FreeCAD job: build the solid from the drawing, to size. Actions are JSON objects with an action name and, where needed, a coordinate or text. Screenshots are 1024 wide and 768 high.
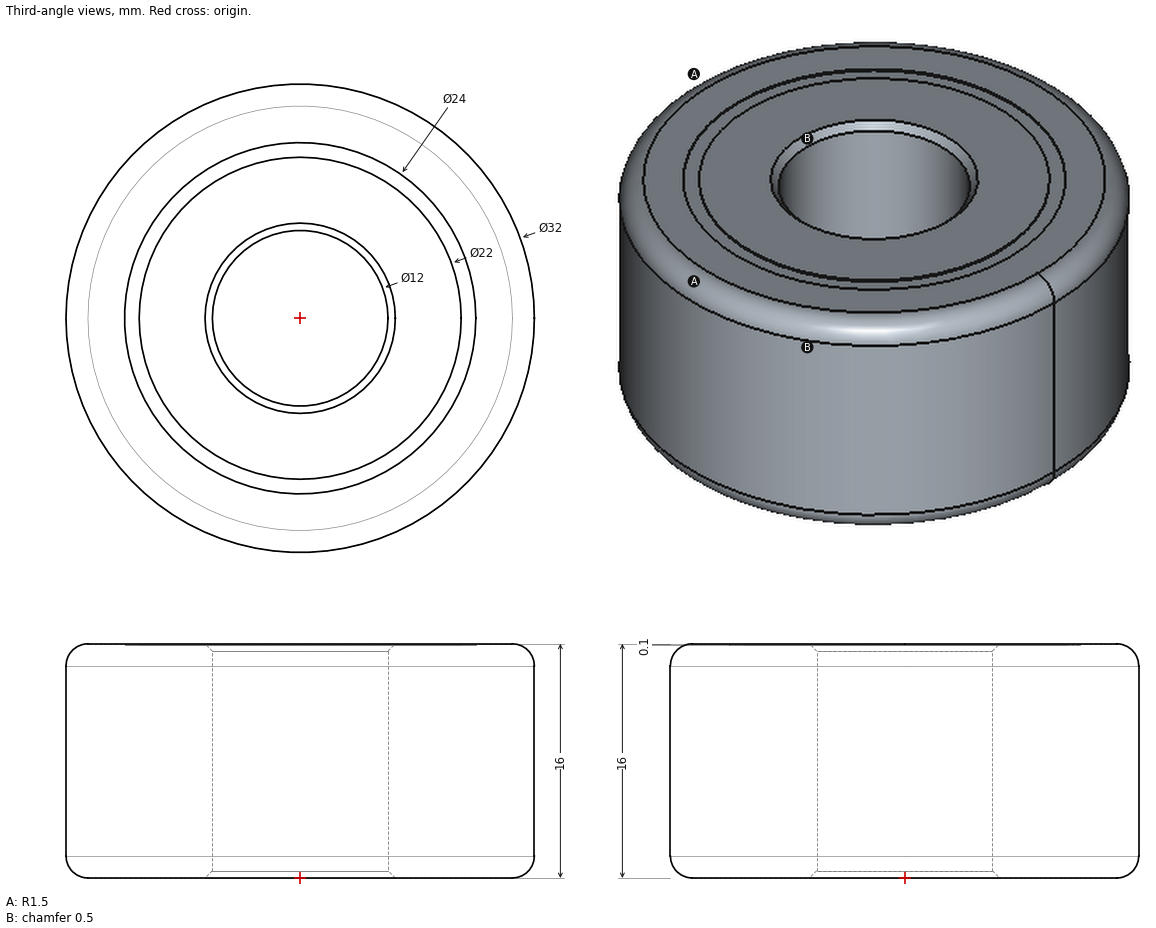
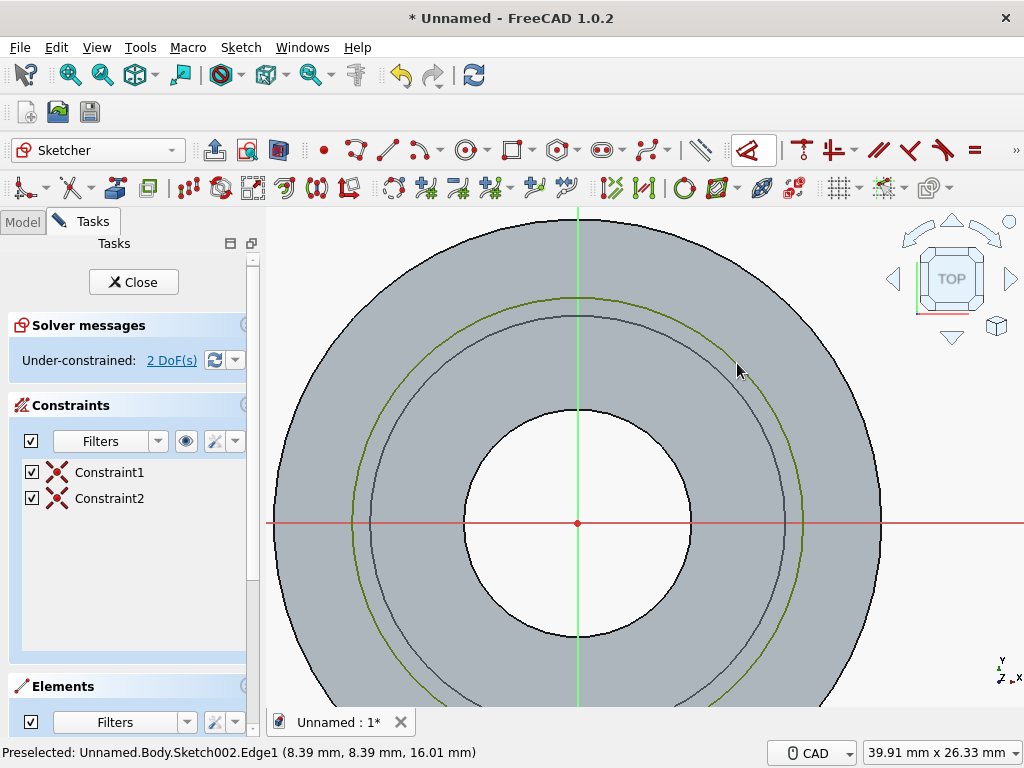
{"action": "key", "text": "k o"}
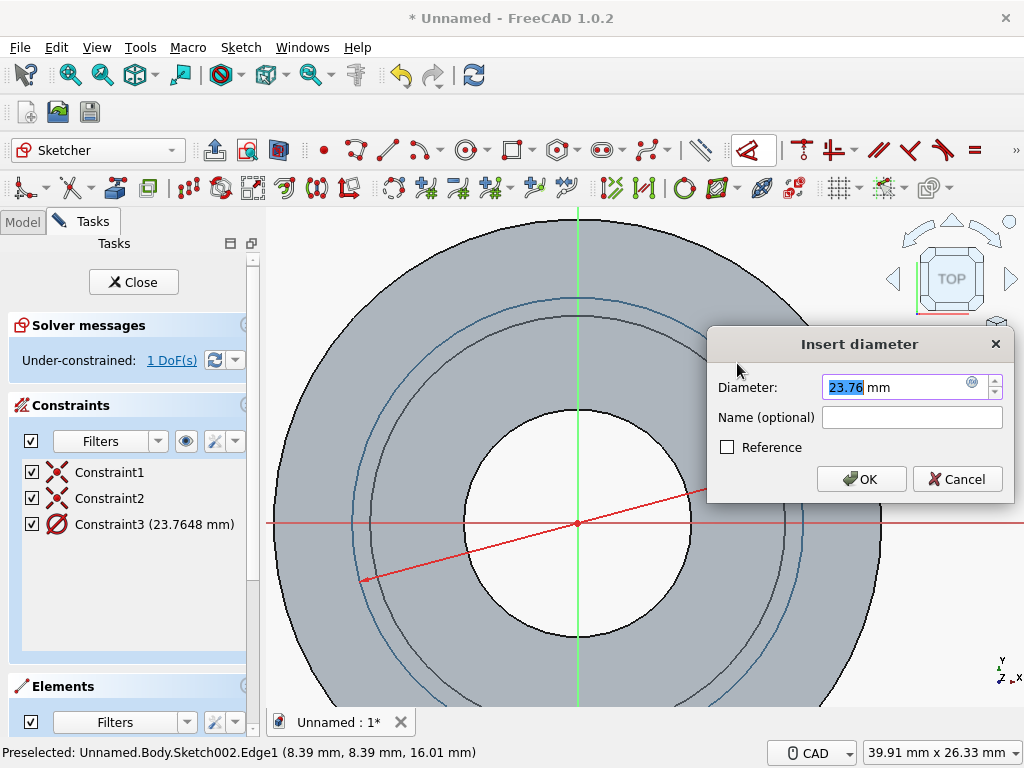
{"action": "type", "text": "24"}
{"action": "key", "text": "Return"}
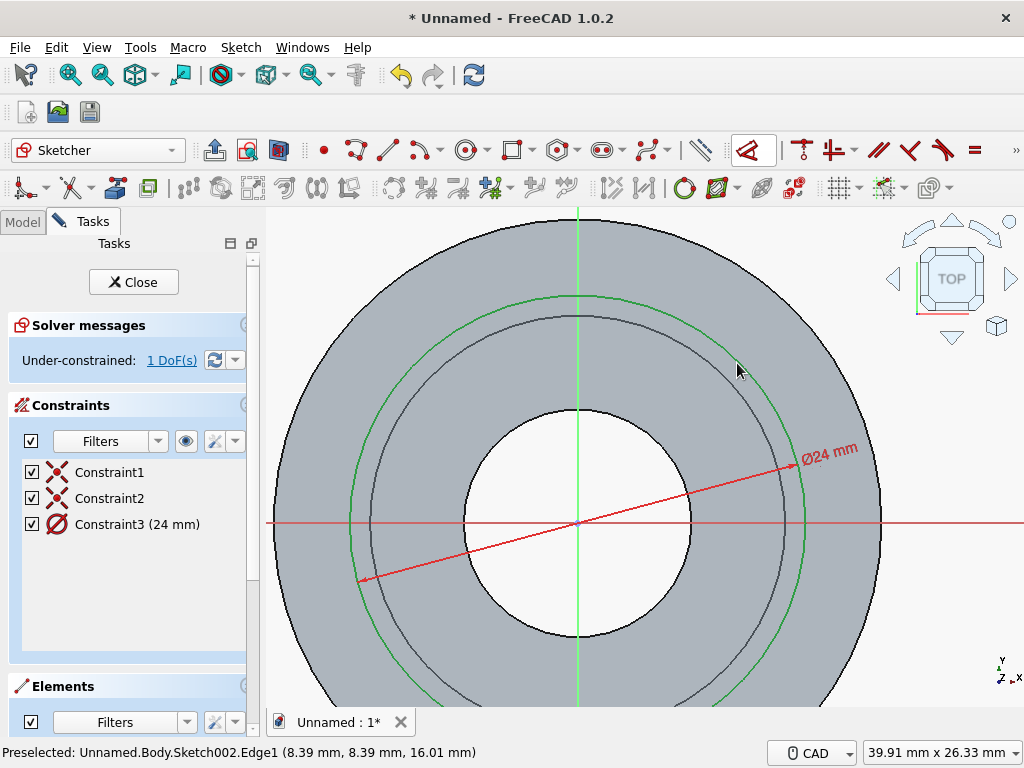
{"action": "left_click", "coordinate": [724, 376]}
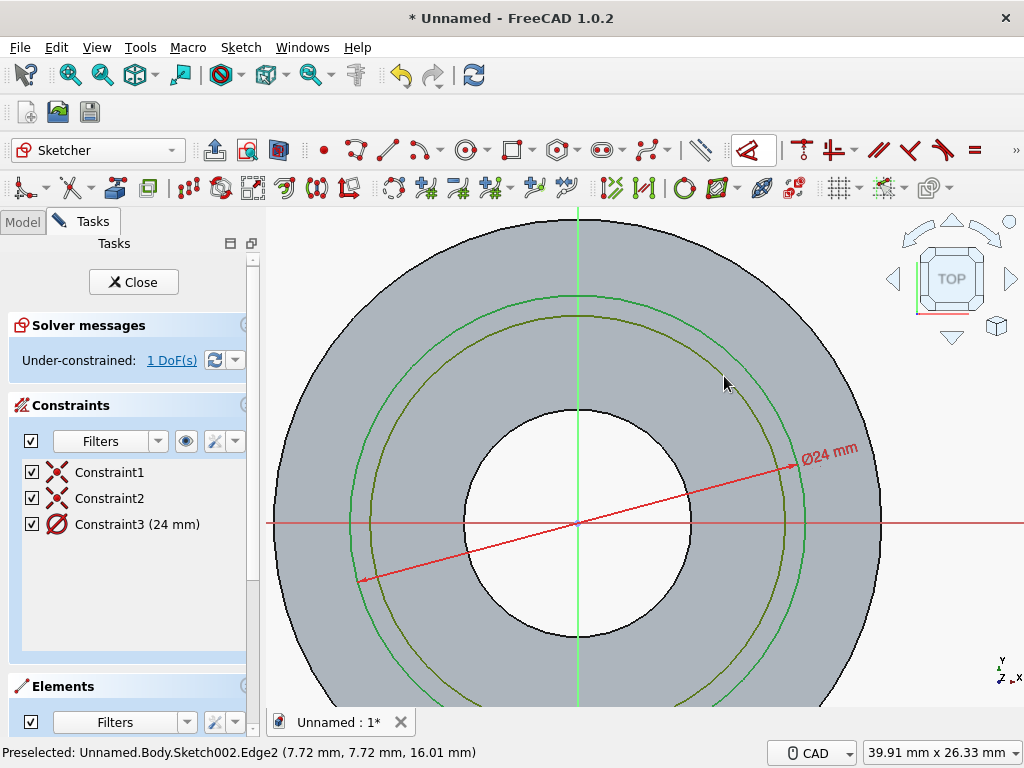
{"action": "left_click", "coordinate": [770, 150]}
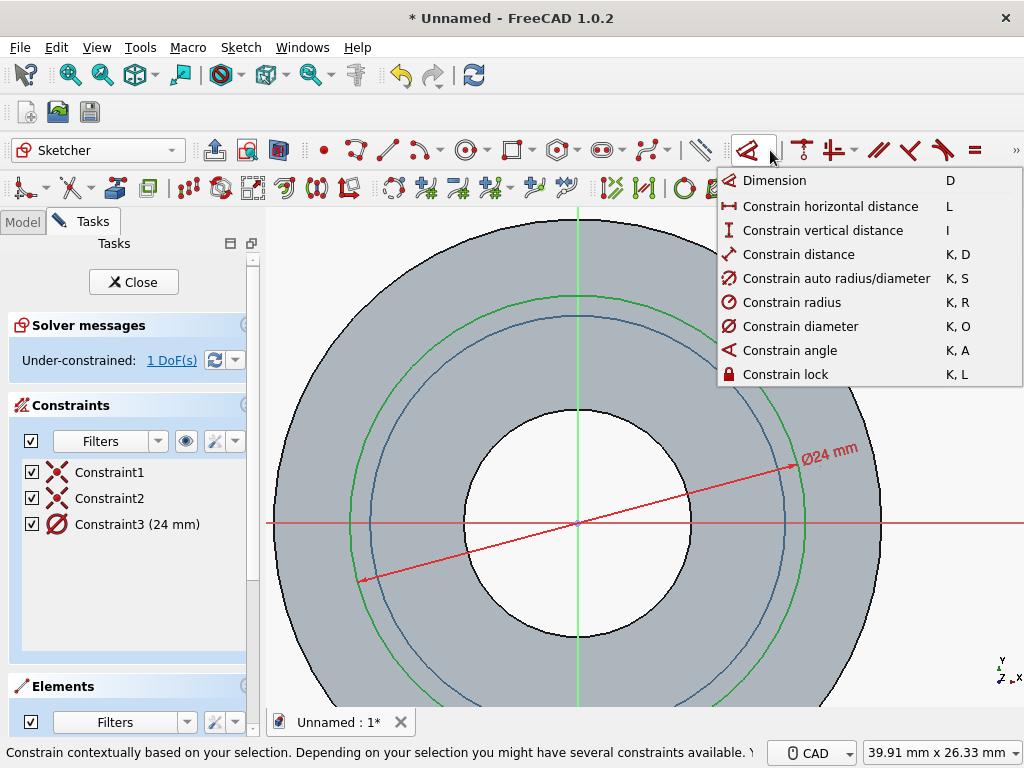
{"action": "left_click", "coordinate": [870, 326]}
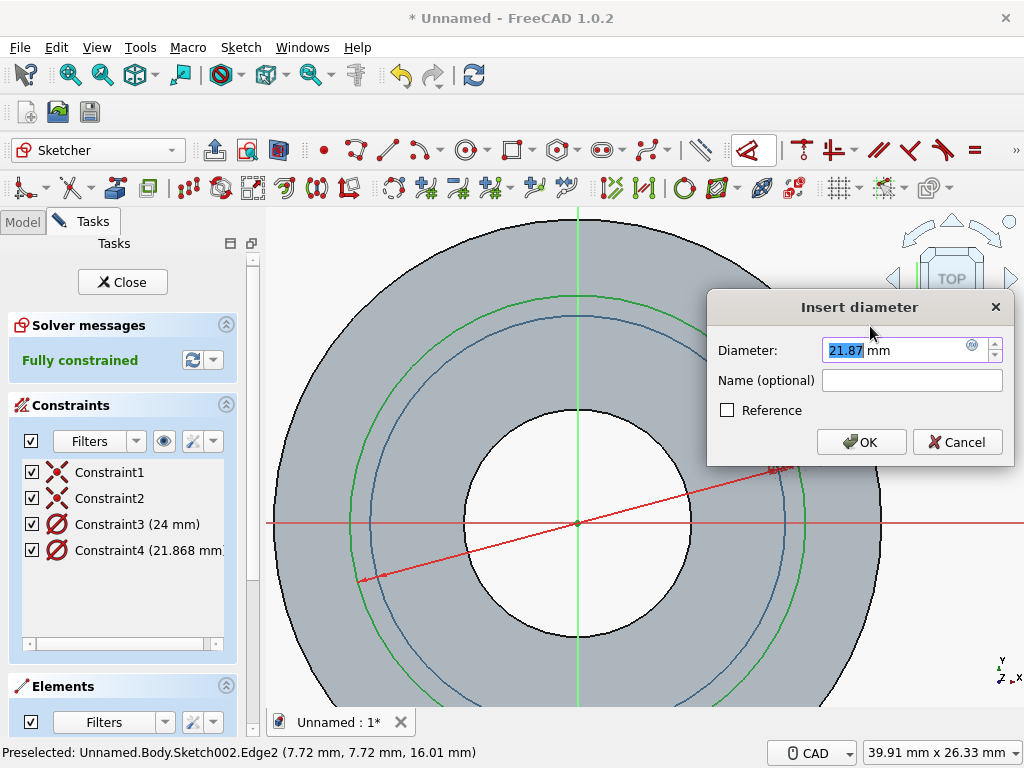
{"action": "type", "text": "22"}
{"action": "key", "text": "Return"}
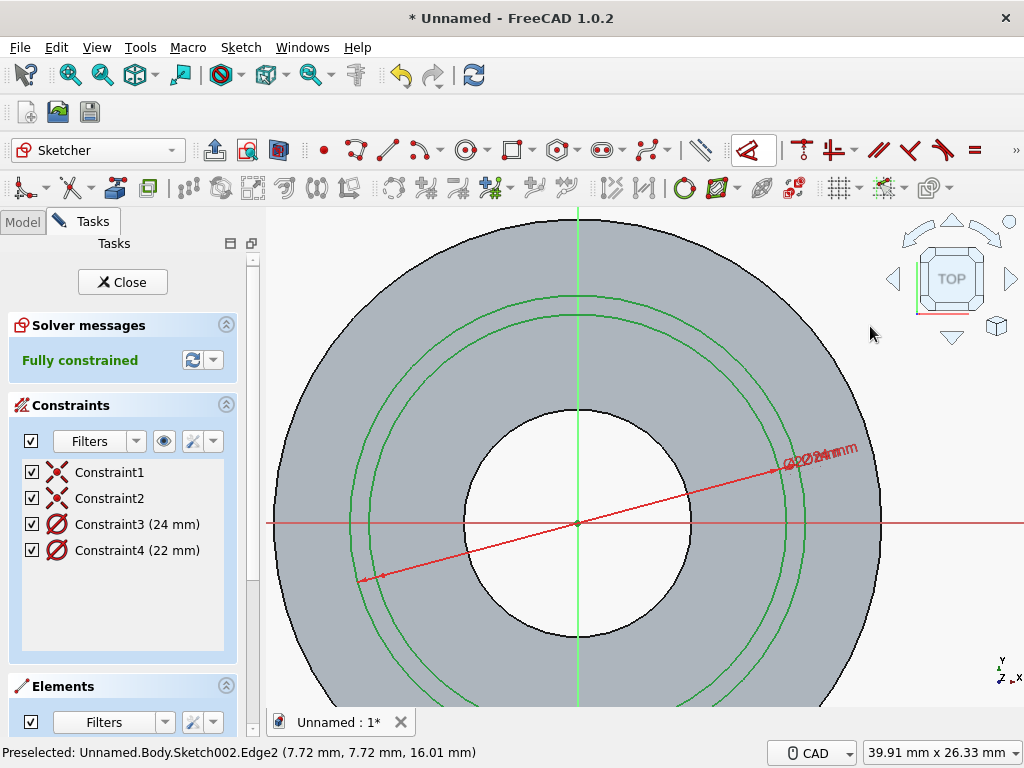
{"action": "left_click", "coordinate": [123, 282]}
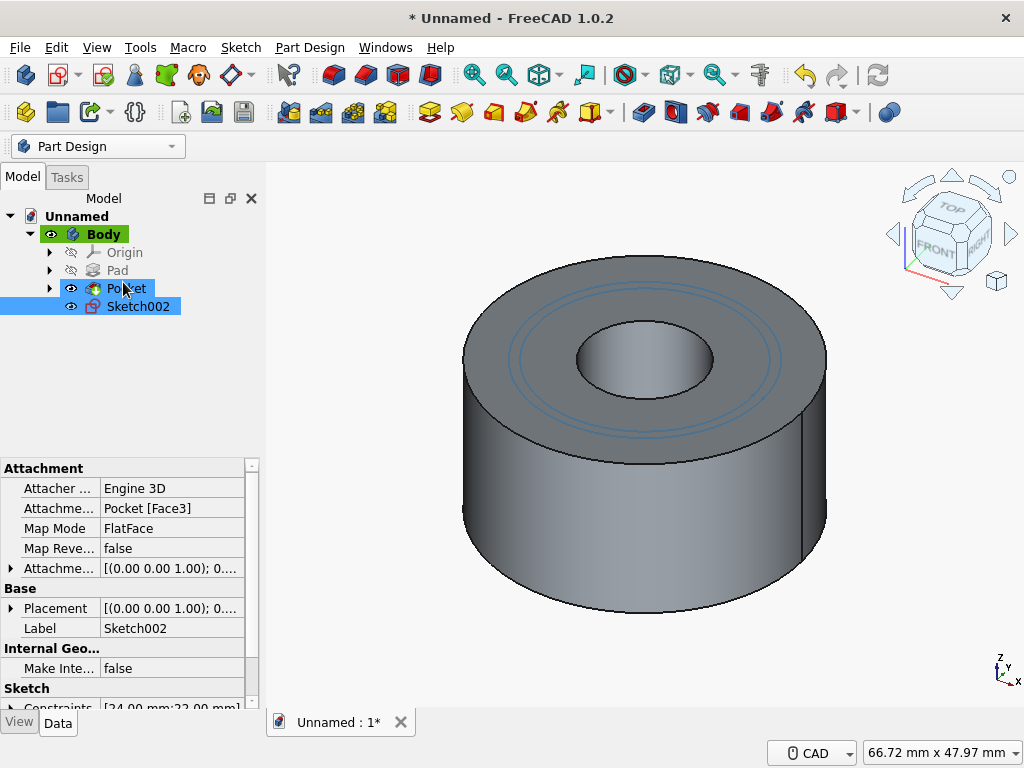
{"action": "left_click", "coordinate": [644, 112]}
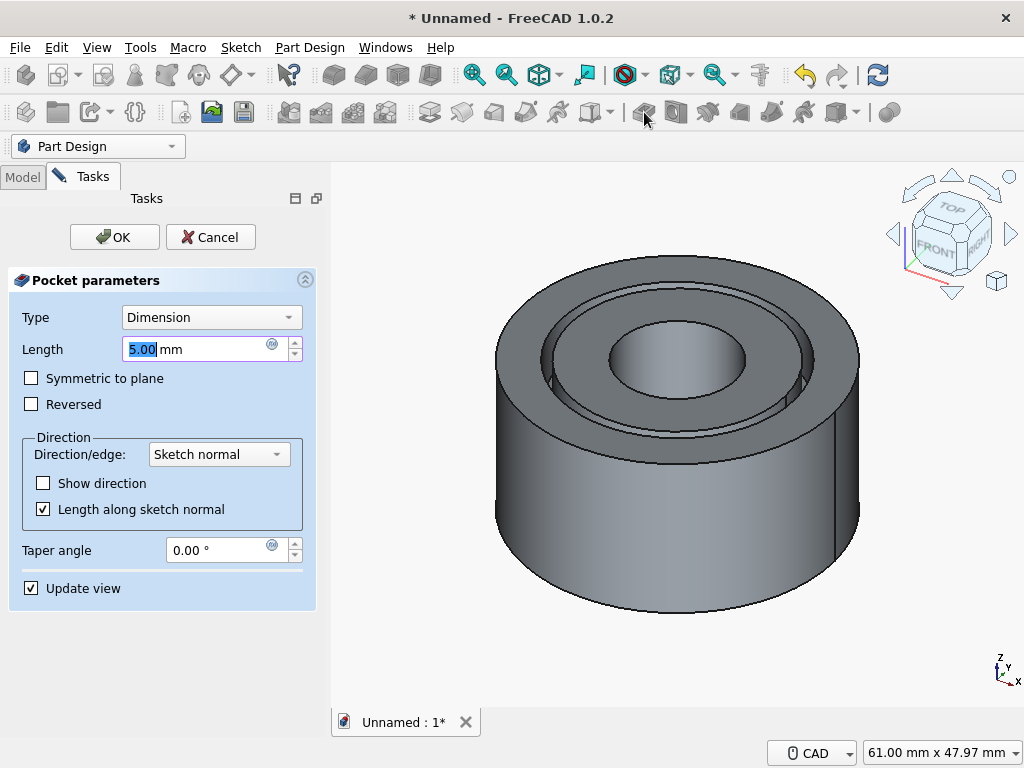
{"action": "type", "text": "0.1"}
{"action": "key", "text": "Tab"}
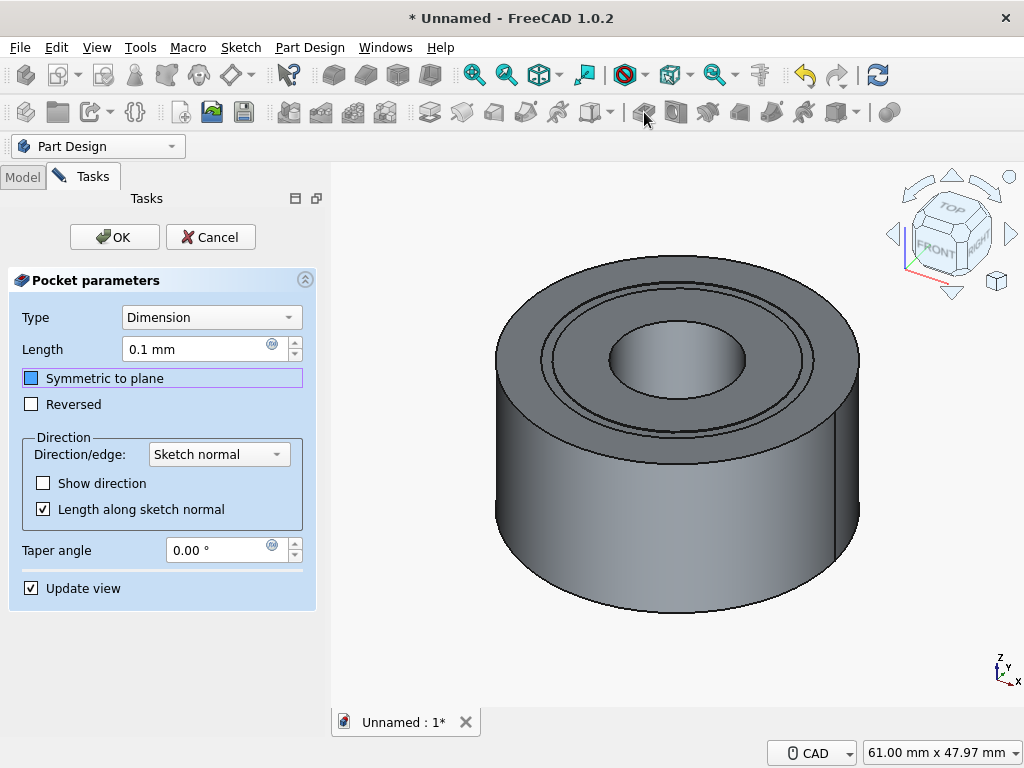
{"action": "left_click", "coordinate": [115, 237]}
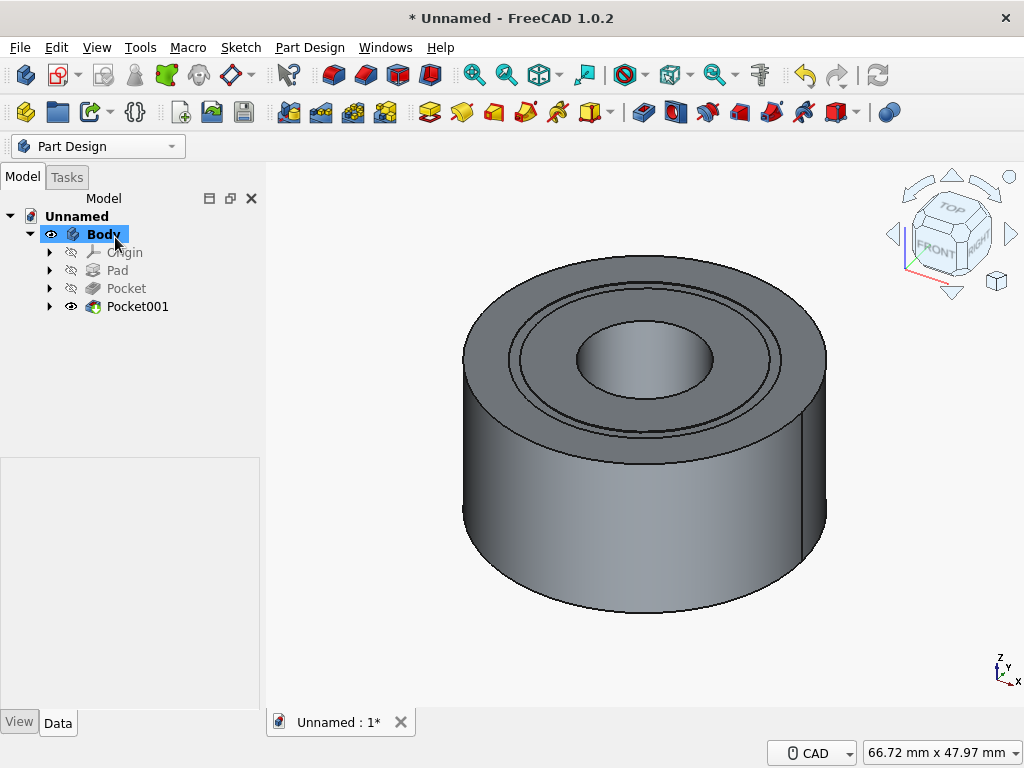
{"action": "left_click", "coordinate": [464, 370]}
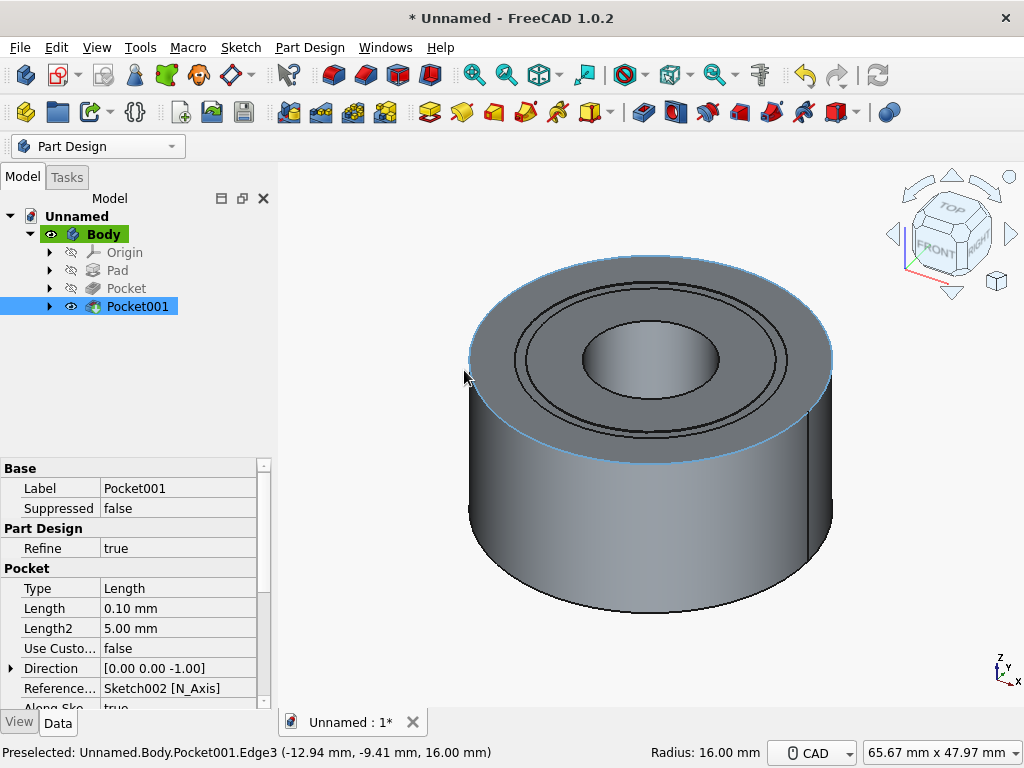
{"action": "key", "text": "0"}